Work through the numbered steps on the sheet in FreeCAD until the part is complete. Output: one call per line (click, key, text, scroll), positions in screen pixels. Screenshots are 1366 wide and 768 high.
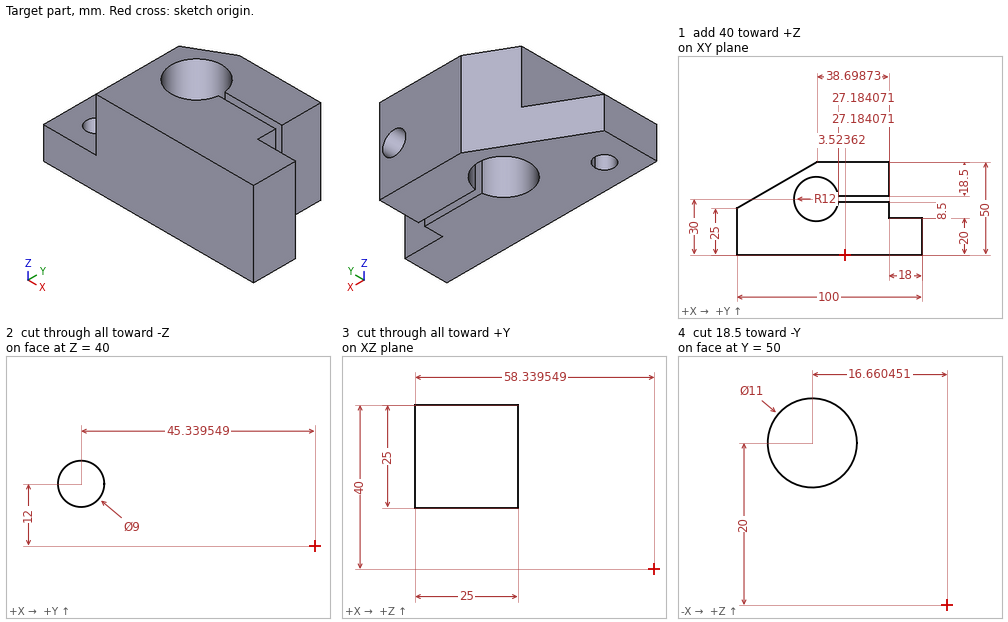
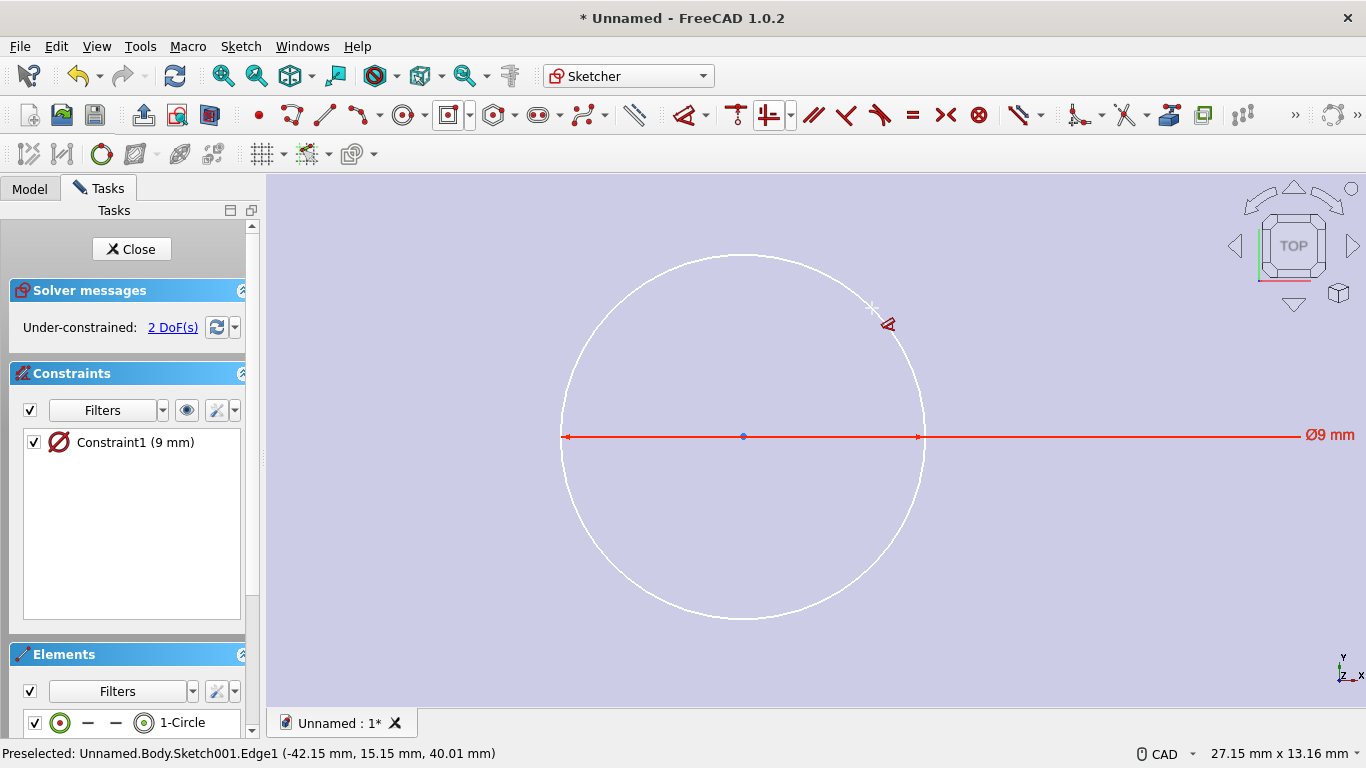
click(743, 437)
click(709, 558)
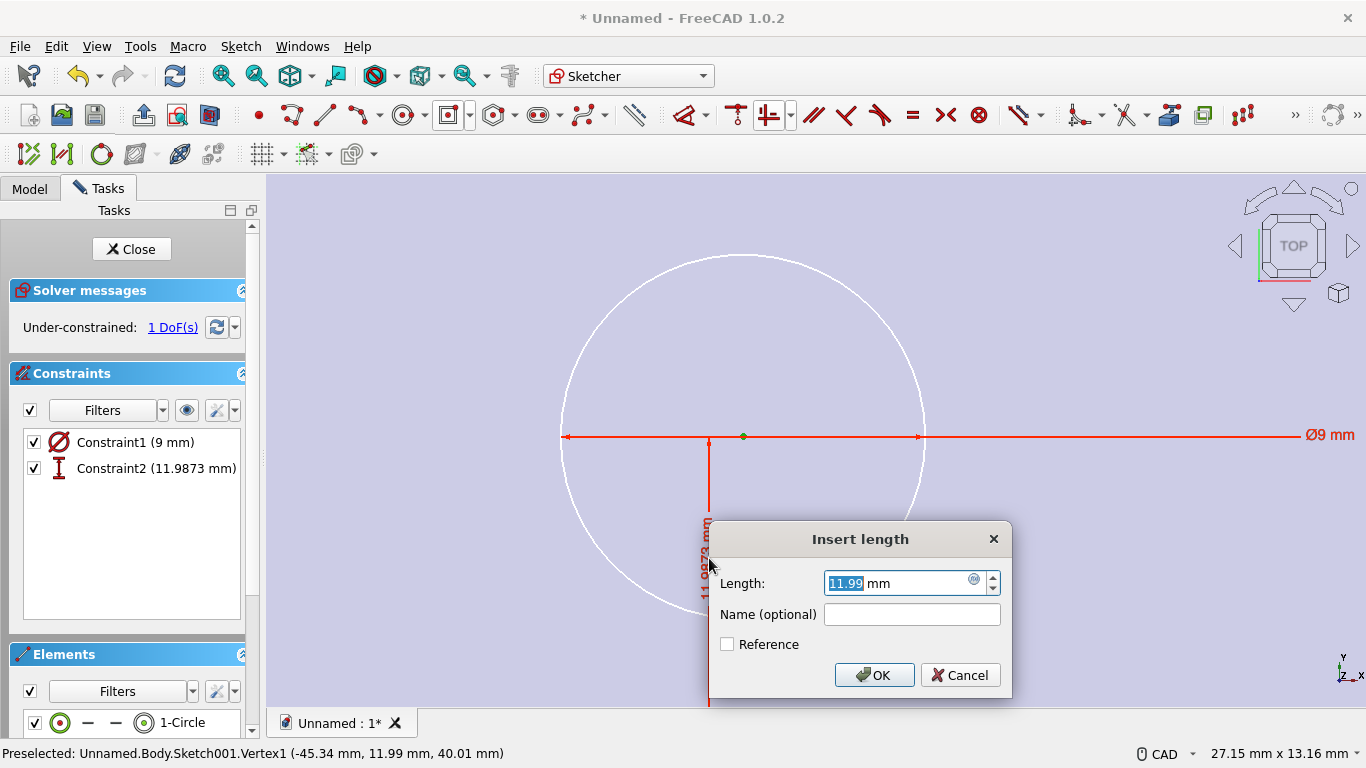
text(12)
key(Return)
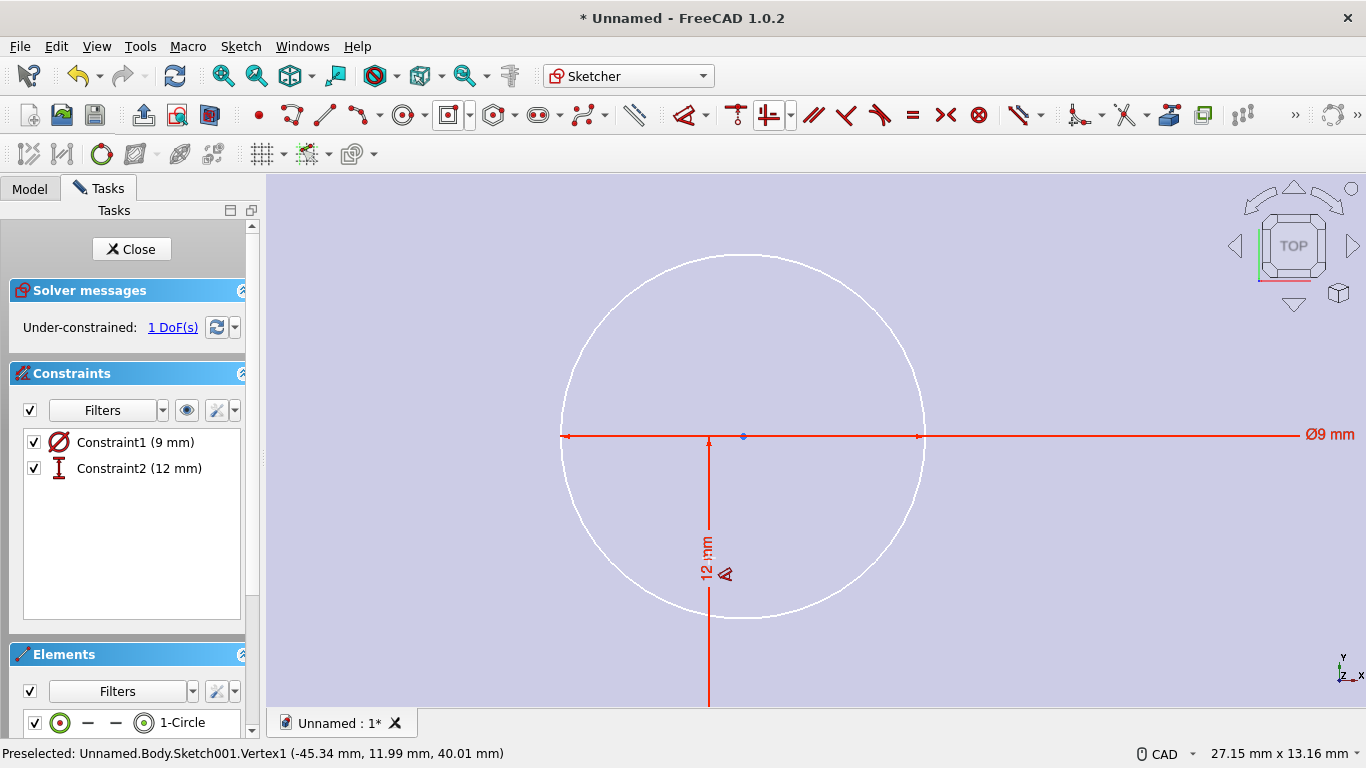
click(743, 436)
click(972, 402)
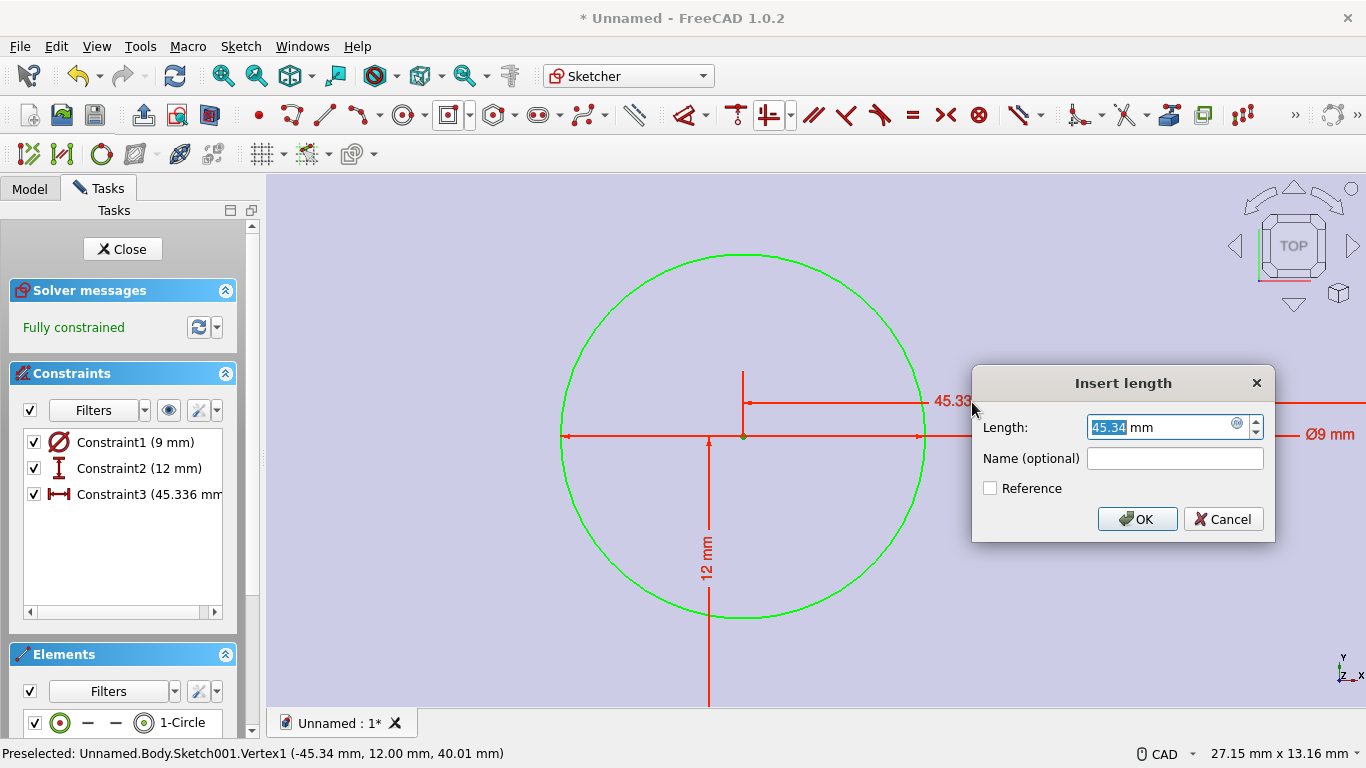
text(45.339549)
key(Return)
key(Escape)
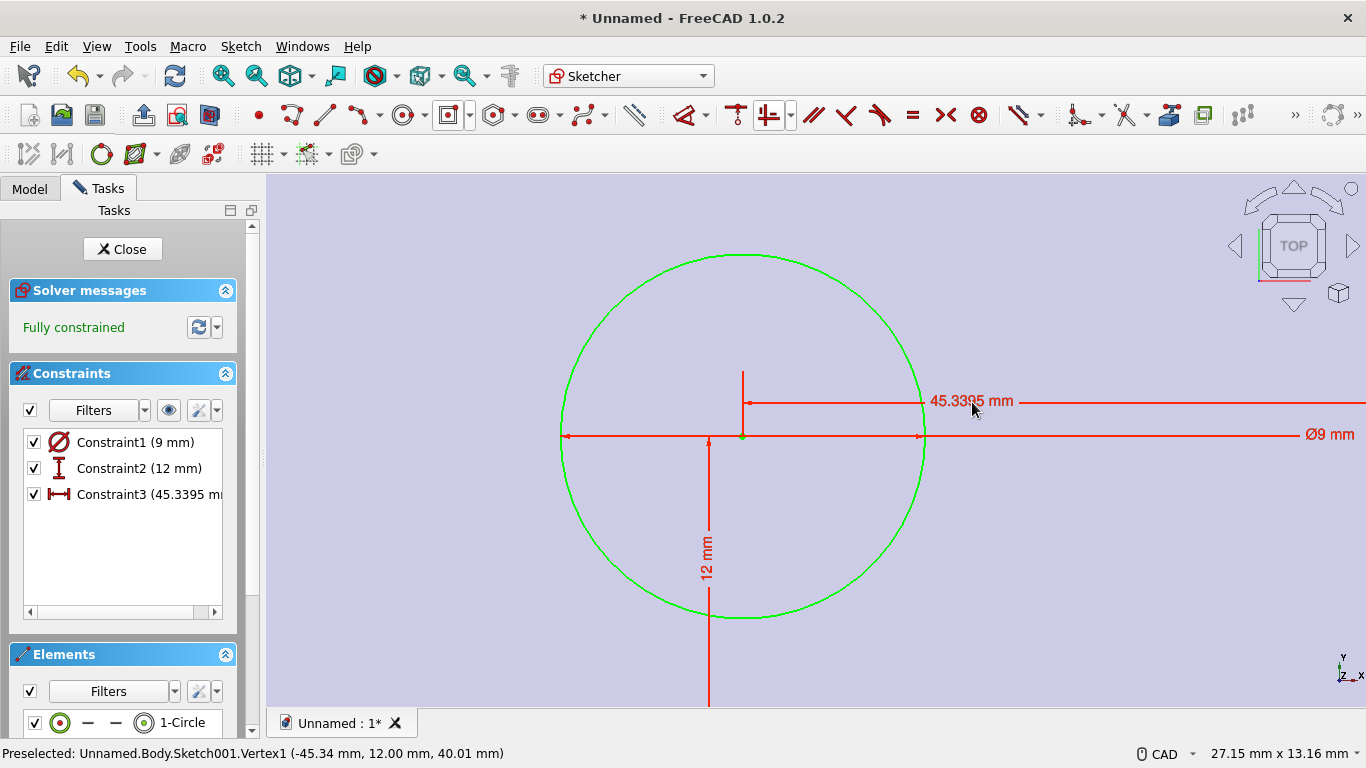
click(123, 249)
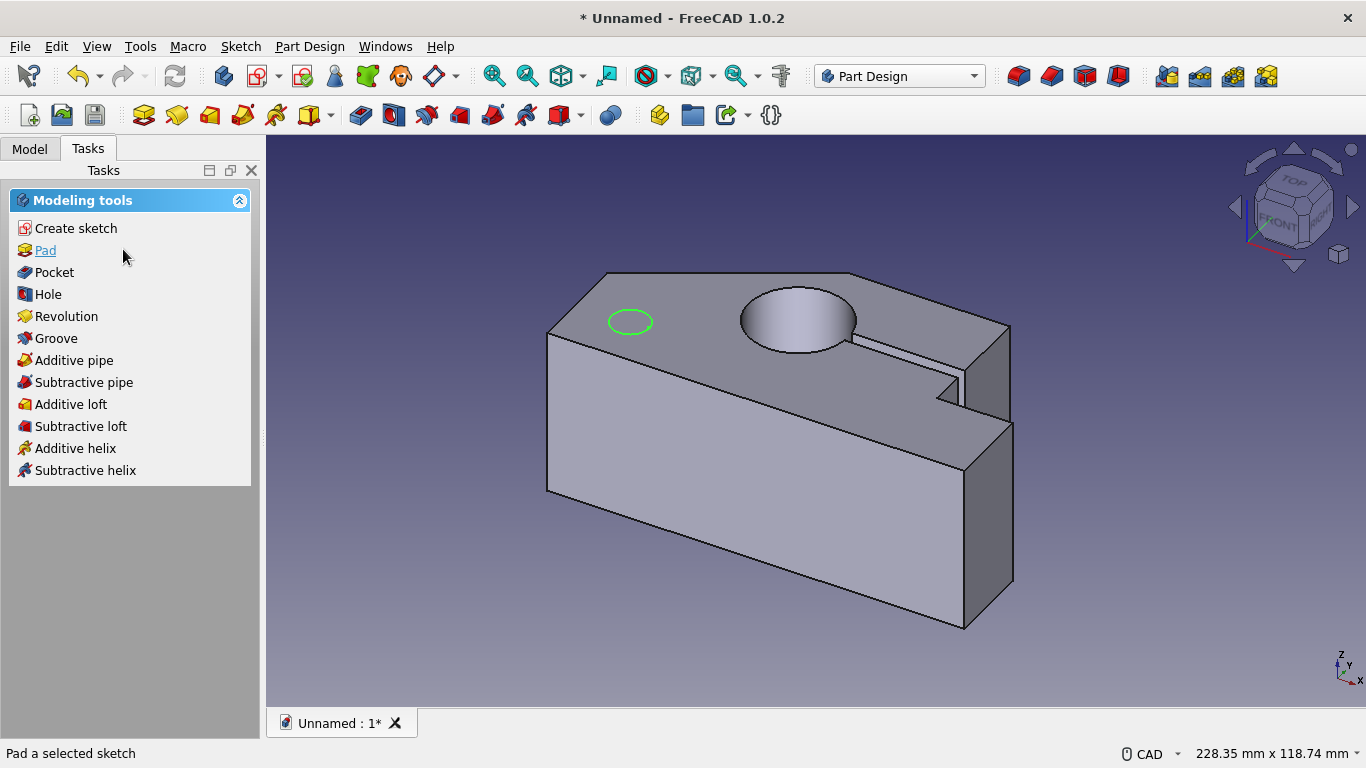
click(361, 116)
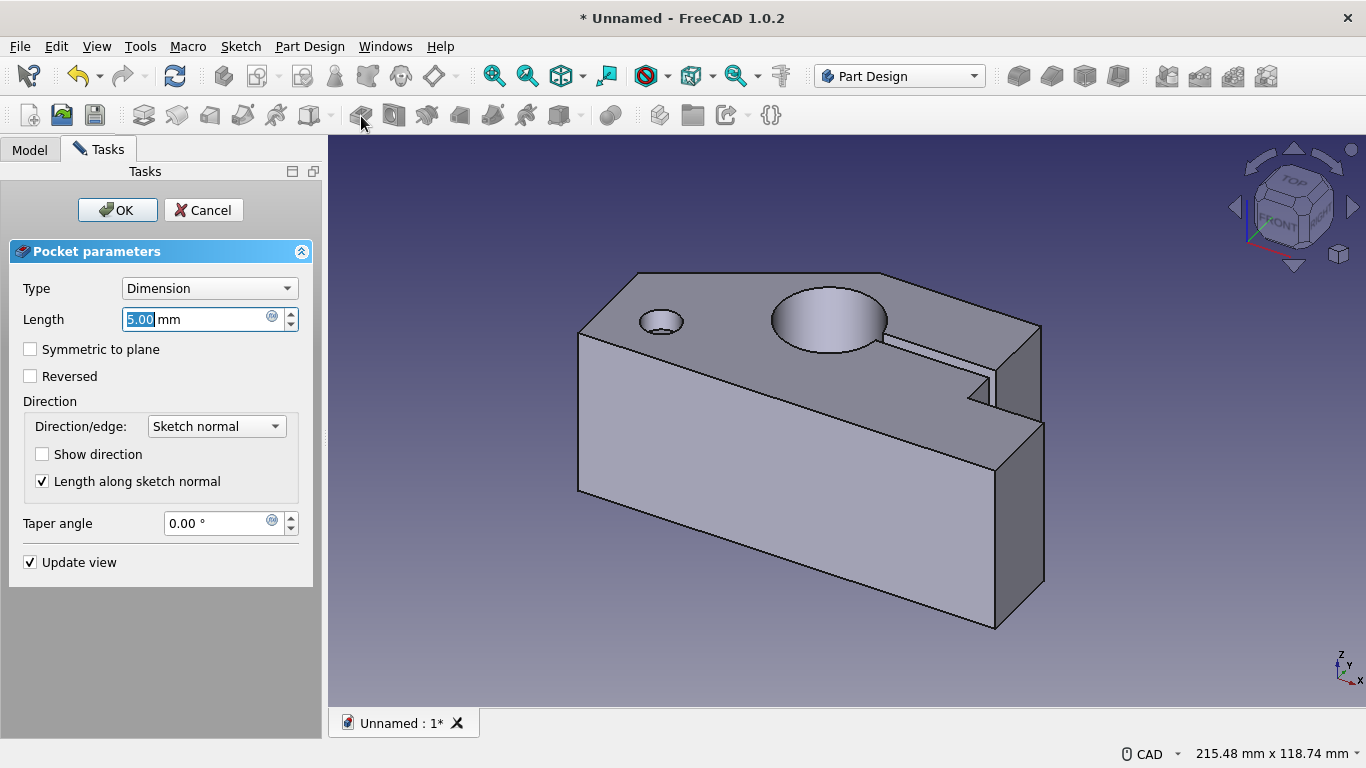
click(210, 288)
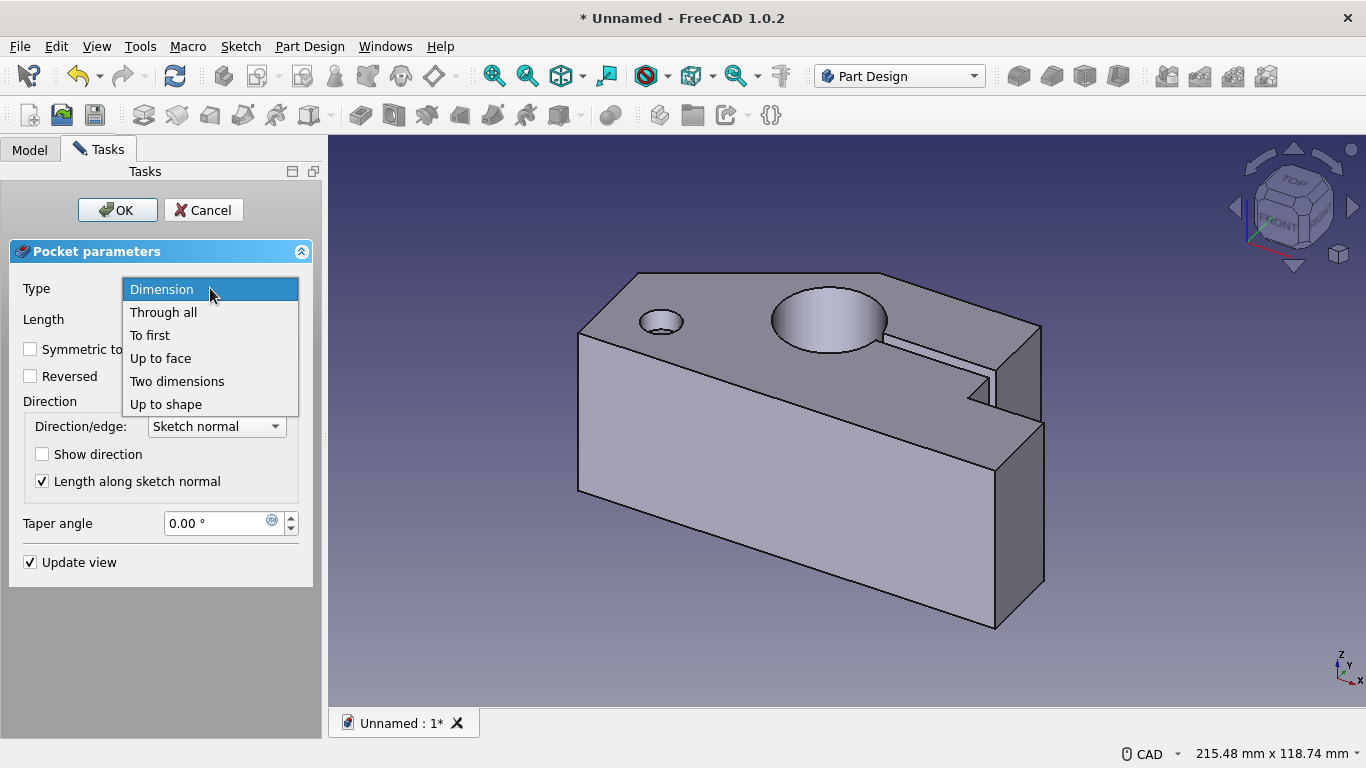
click(208, 312)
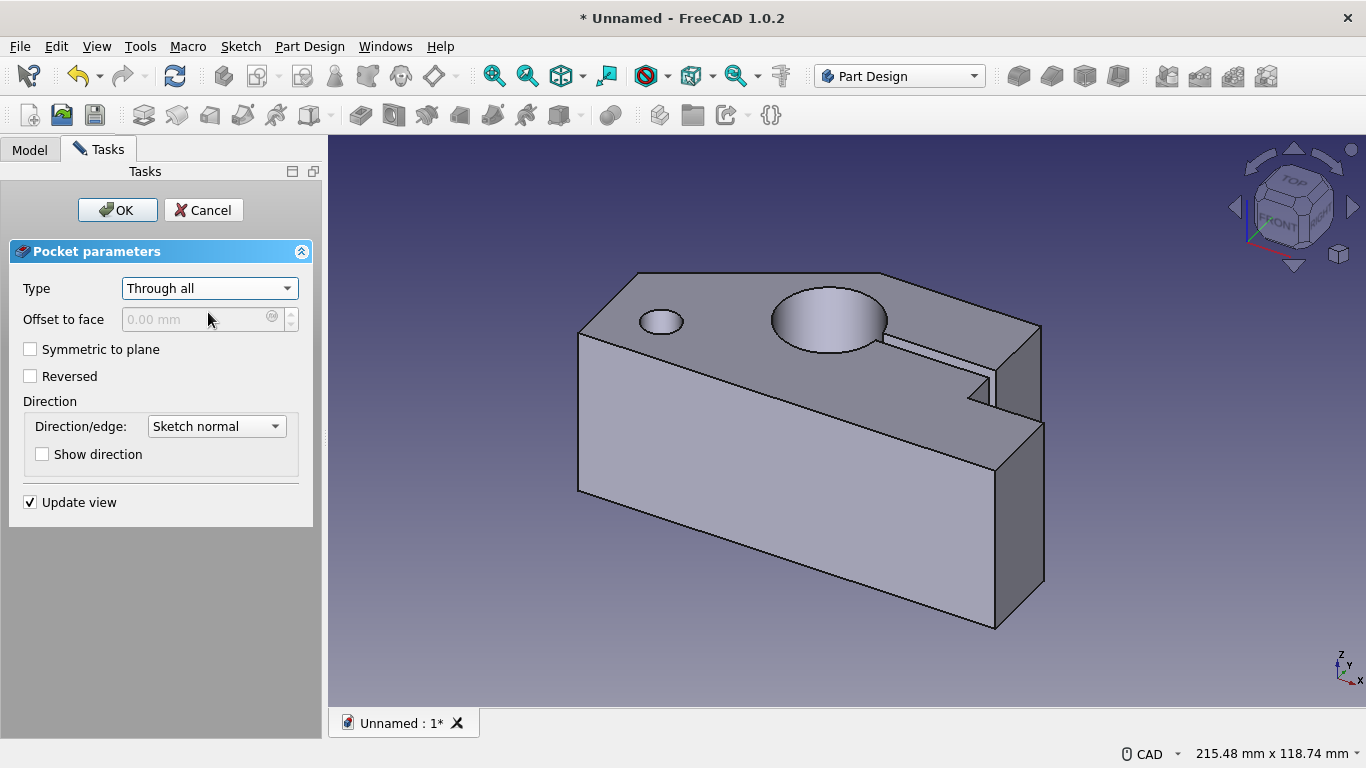
click(118, 210)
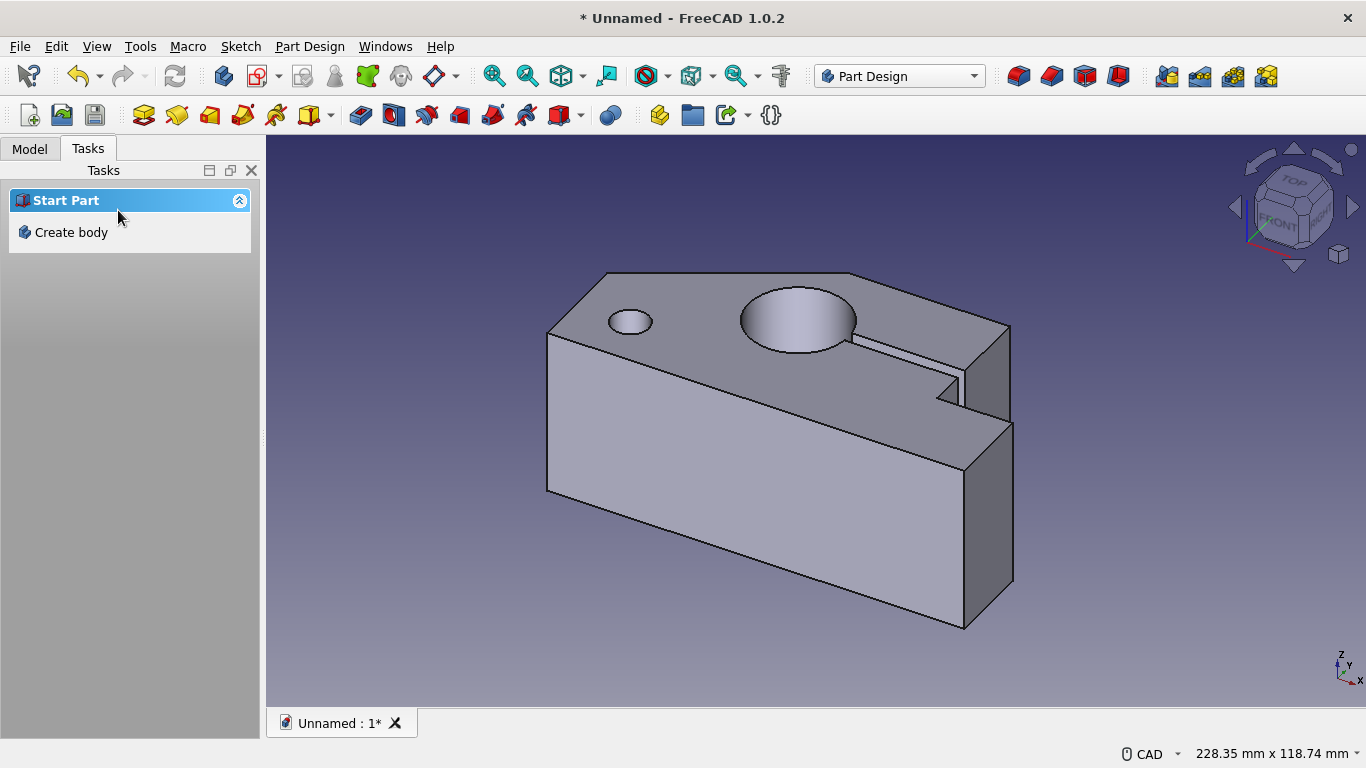
click(256, 76)